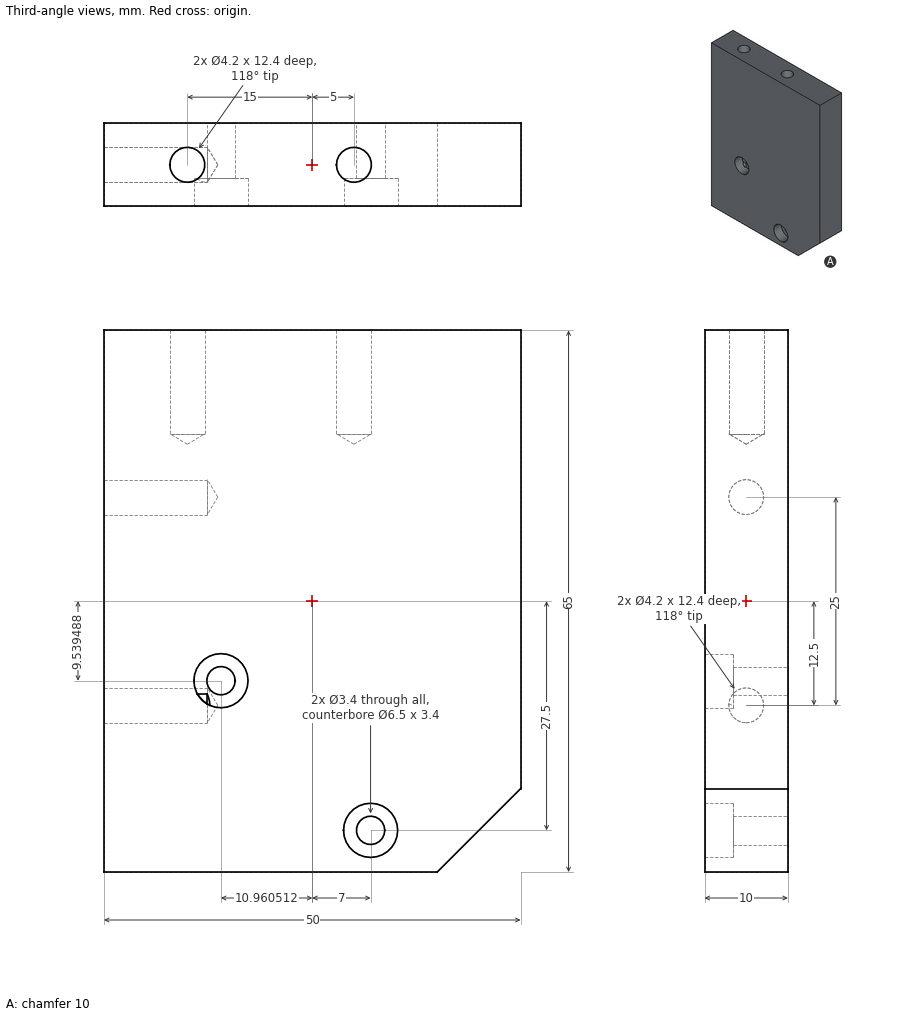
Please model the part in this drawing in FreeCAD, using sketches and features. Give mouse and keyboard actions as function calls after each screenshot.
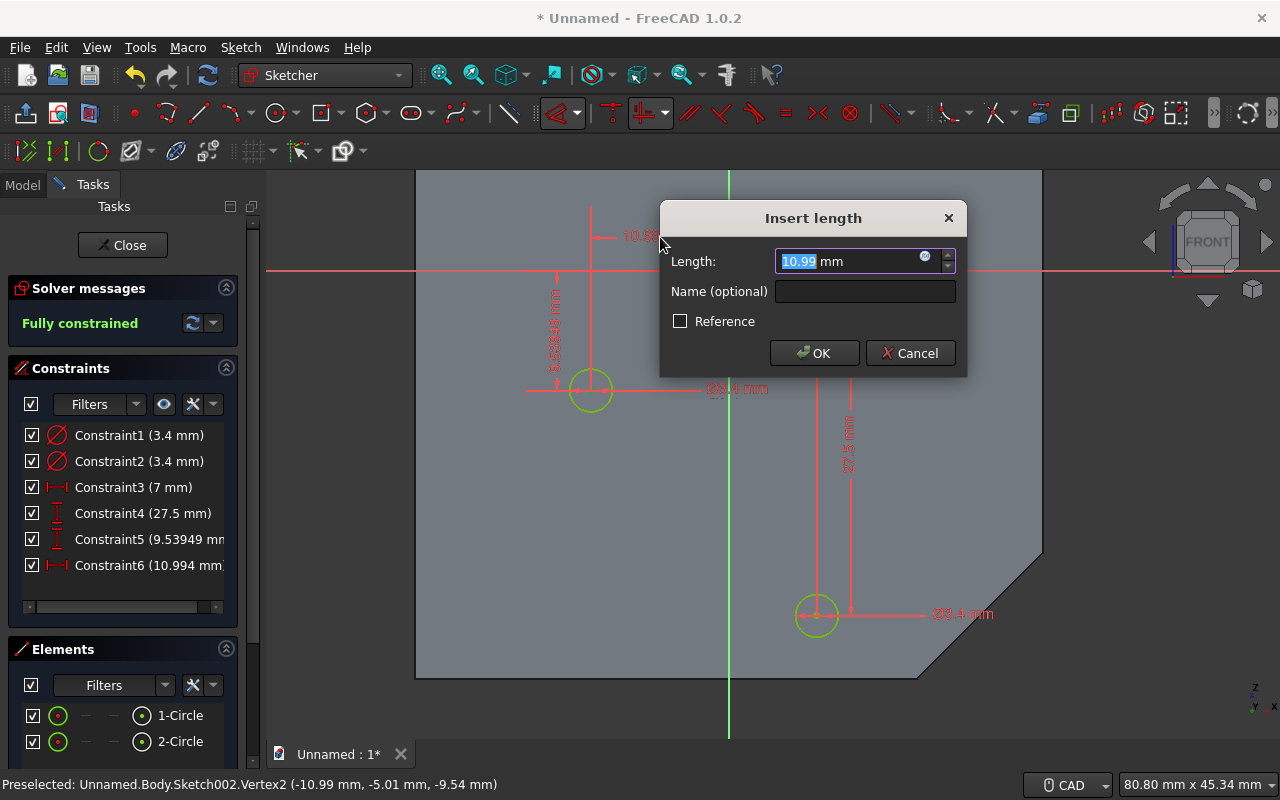
text(10.960512)
key(Return)
key(Escape)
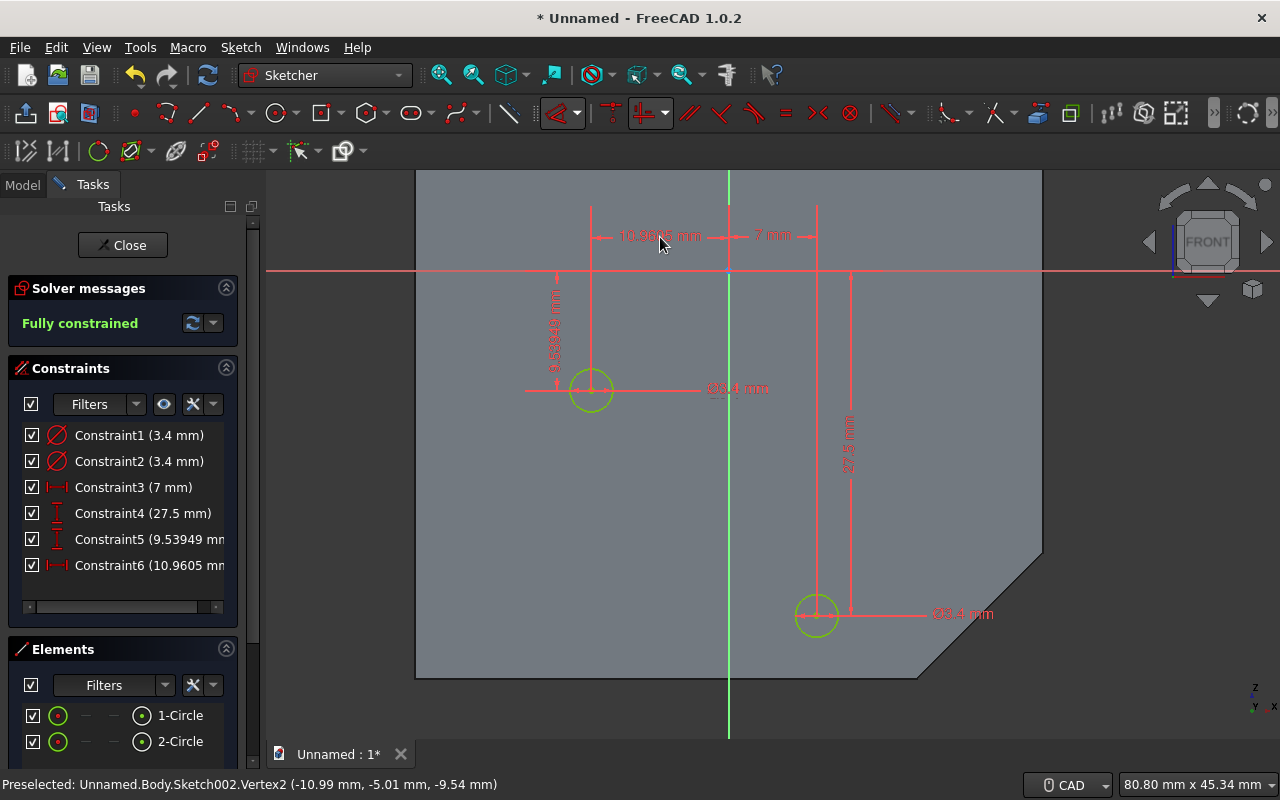
click(123, 245)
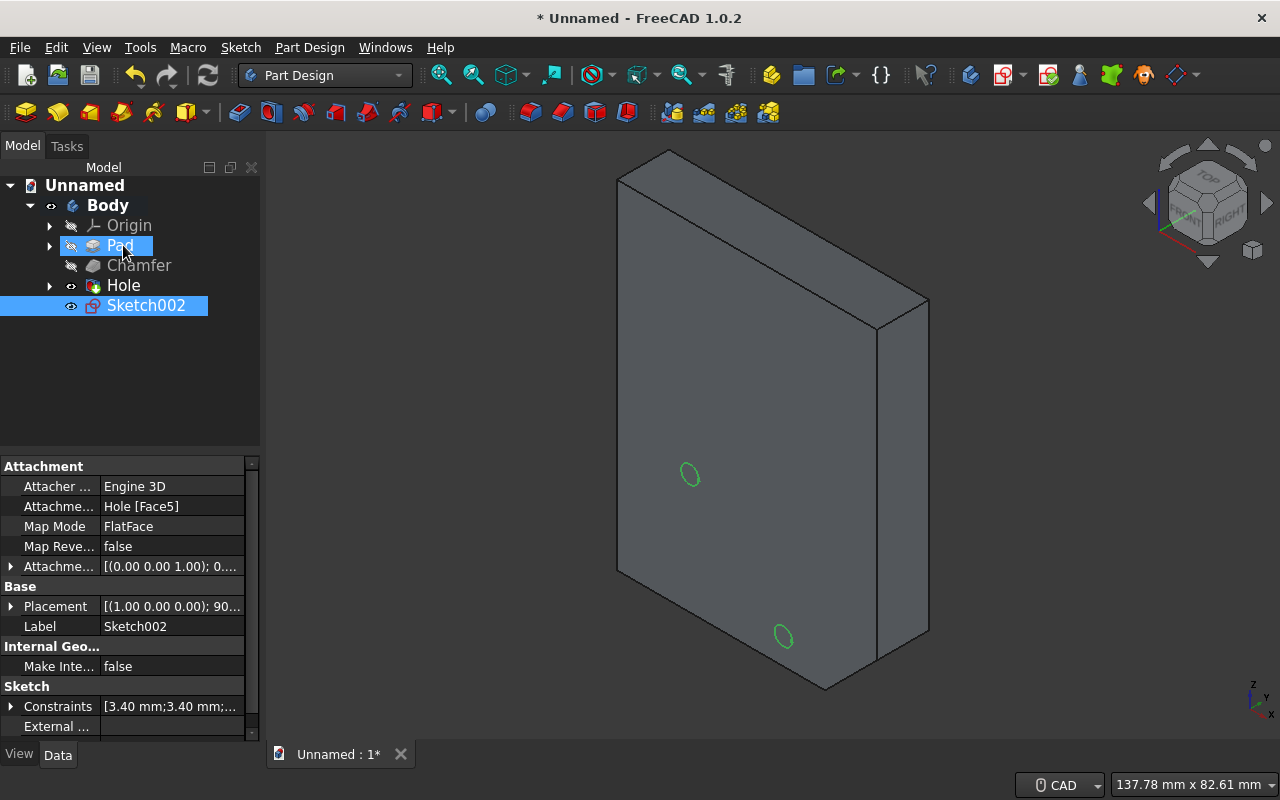
click(272, 112)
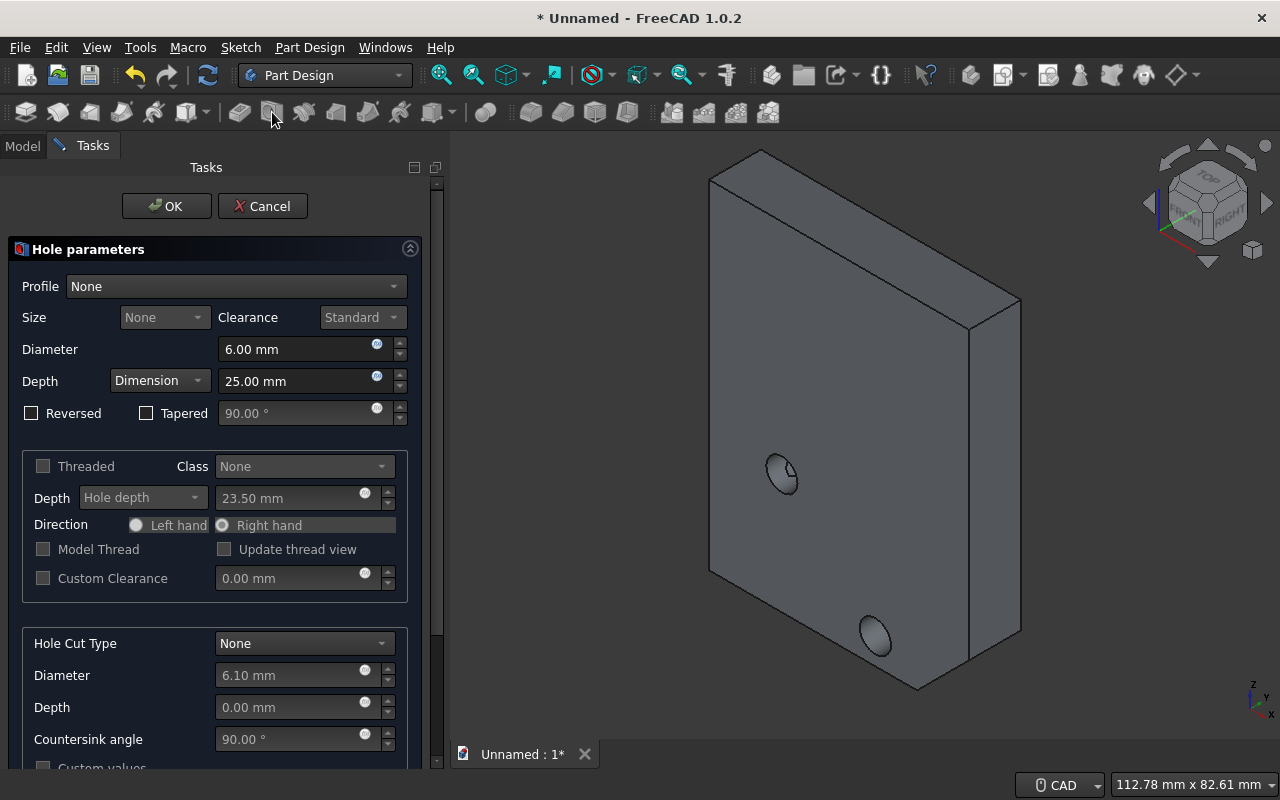
triple_click(305, 349)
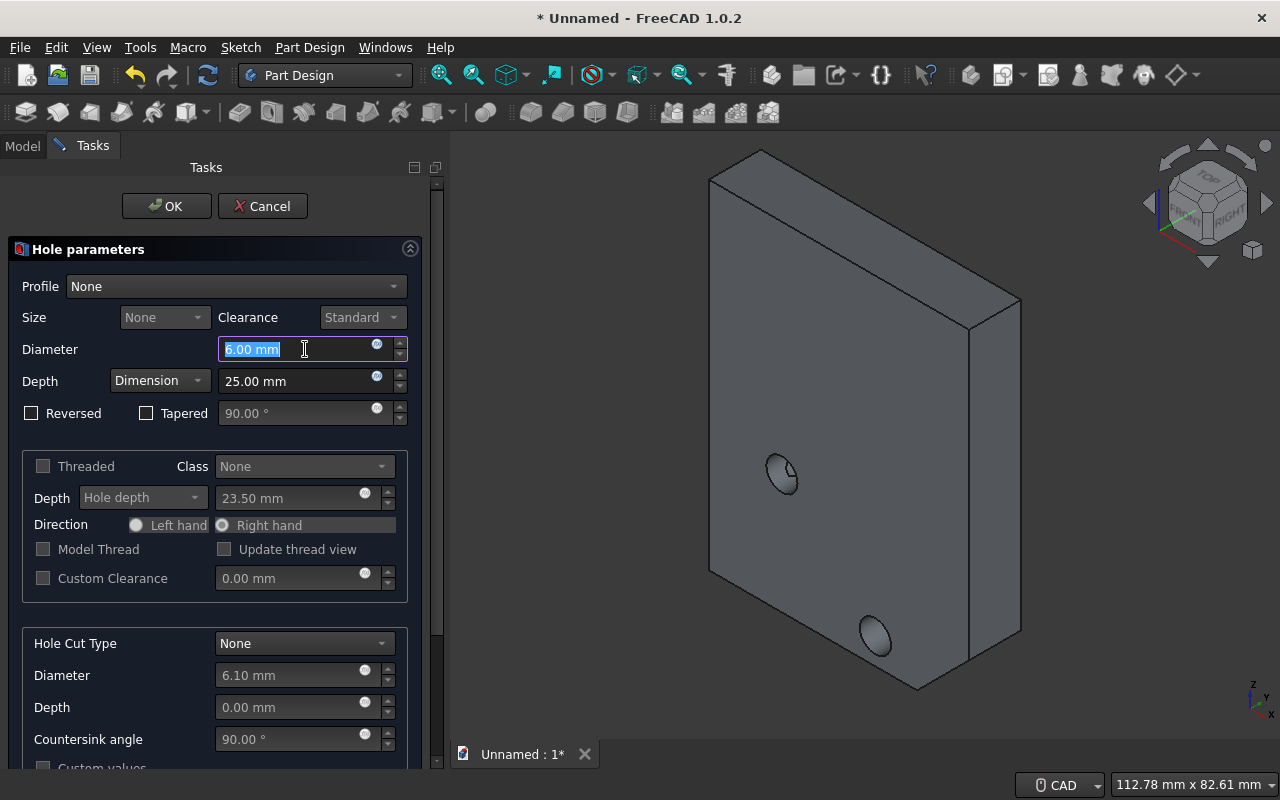
text(3.4)
key(Tab)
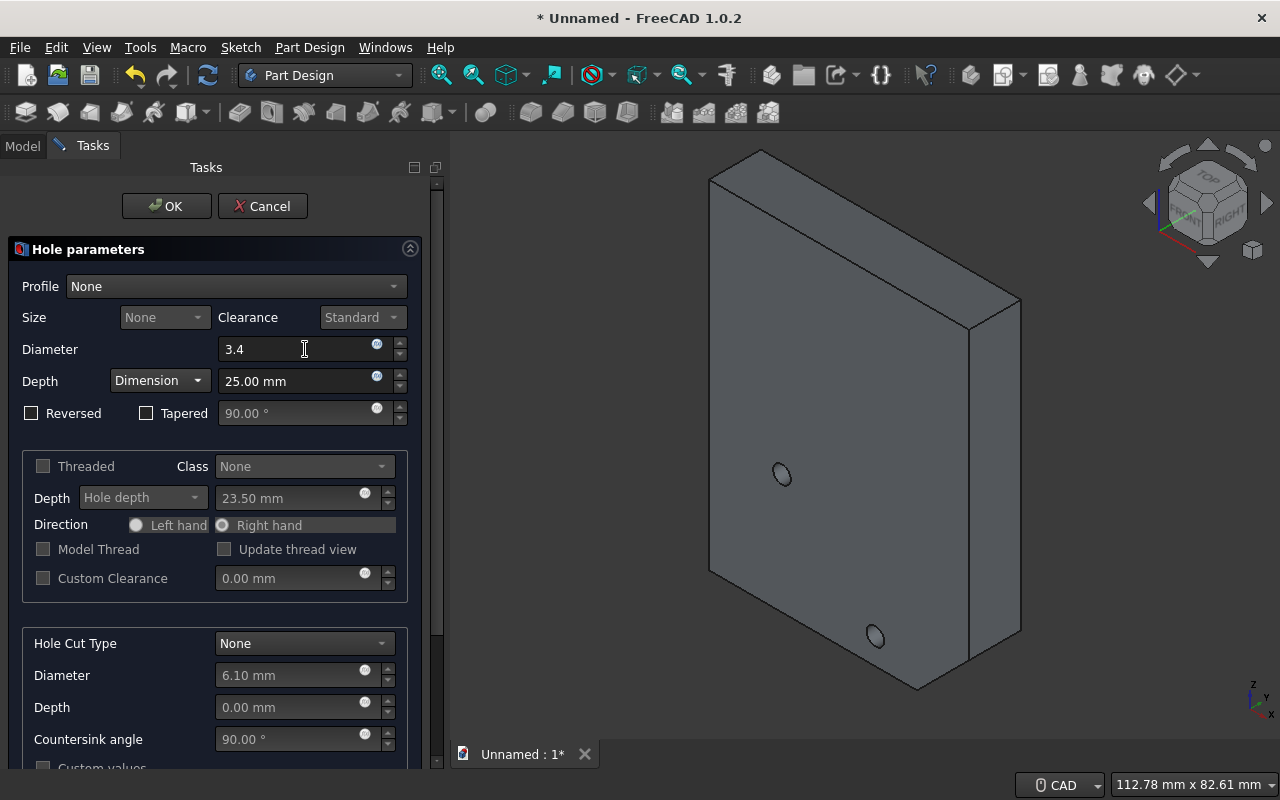
click(161, 380)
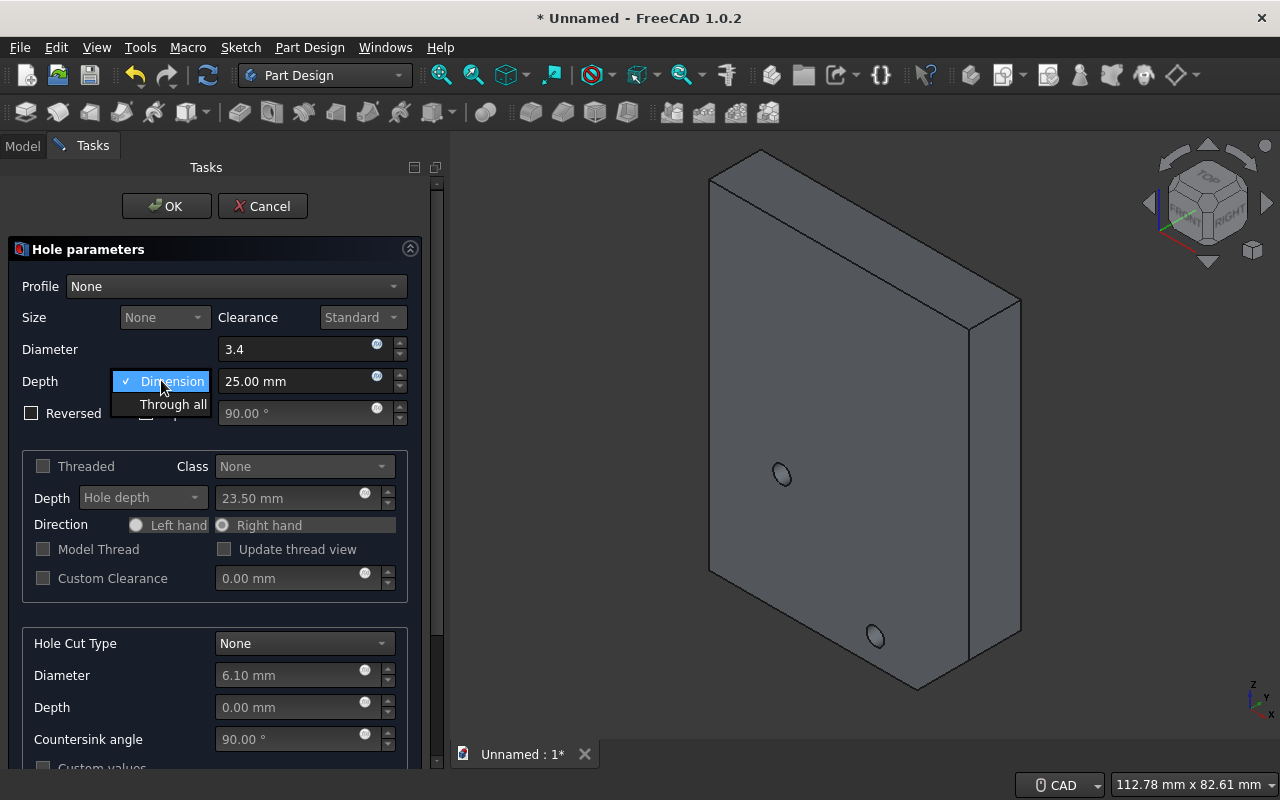
click(160, 404)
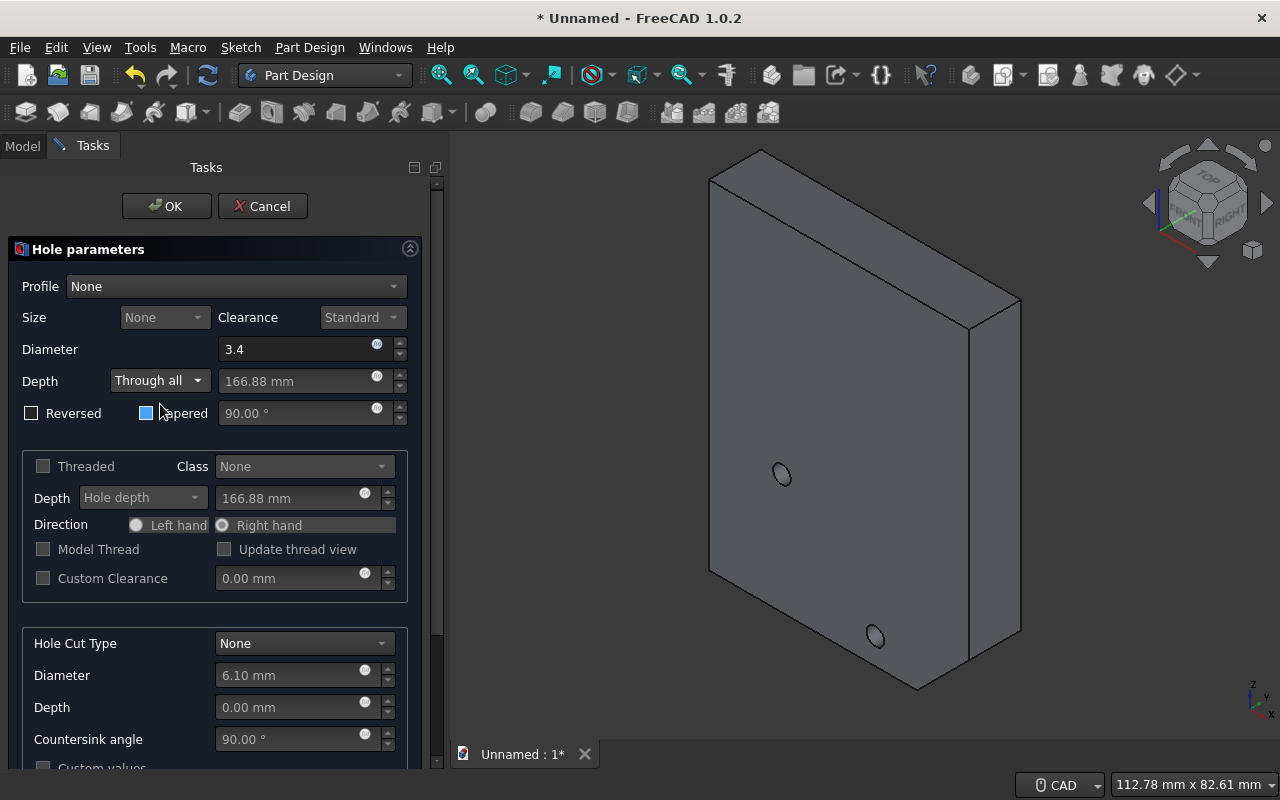
click(306, 644)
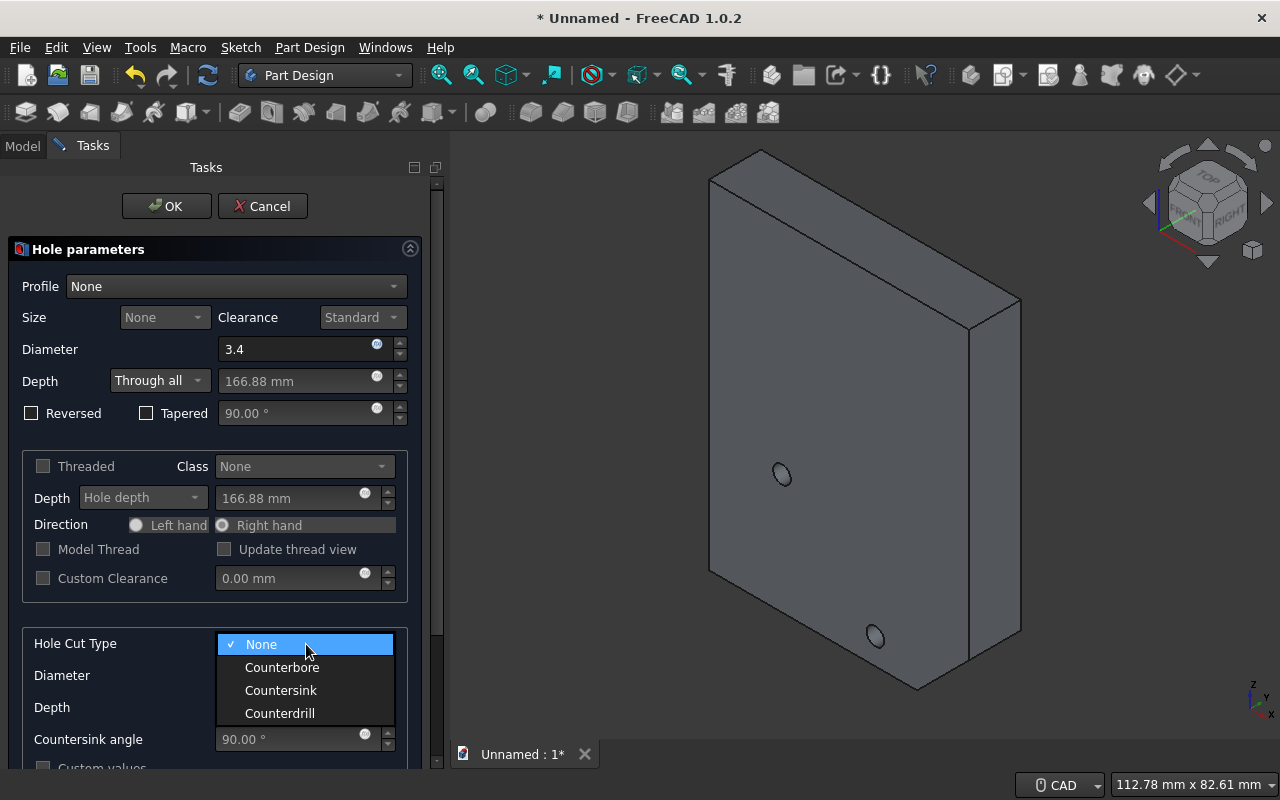
click(304, 668)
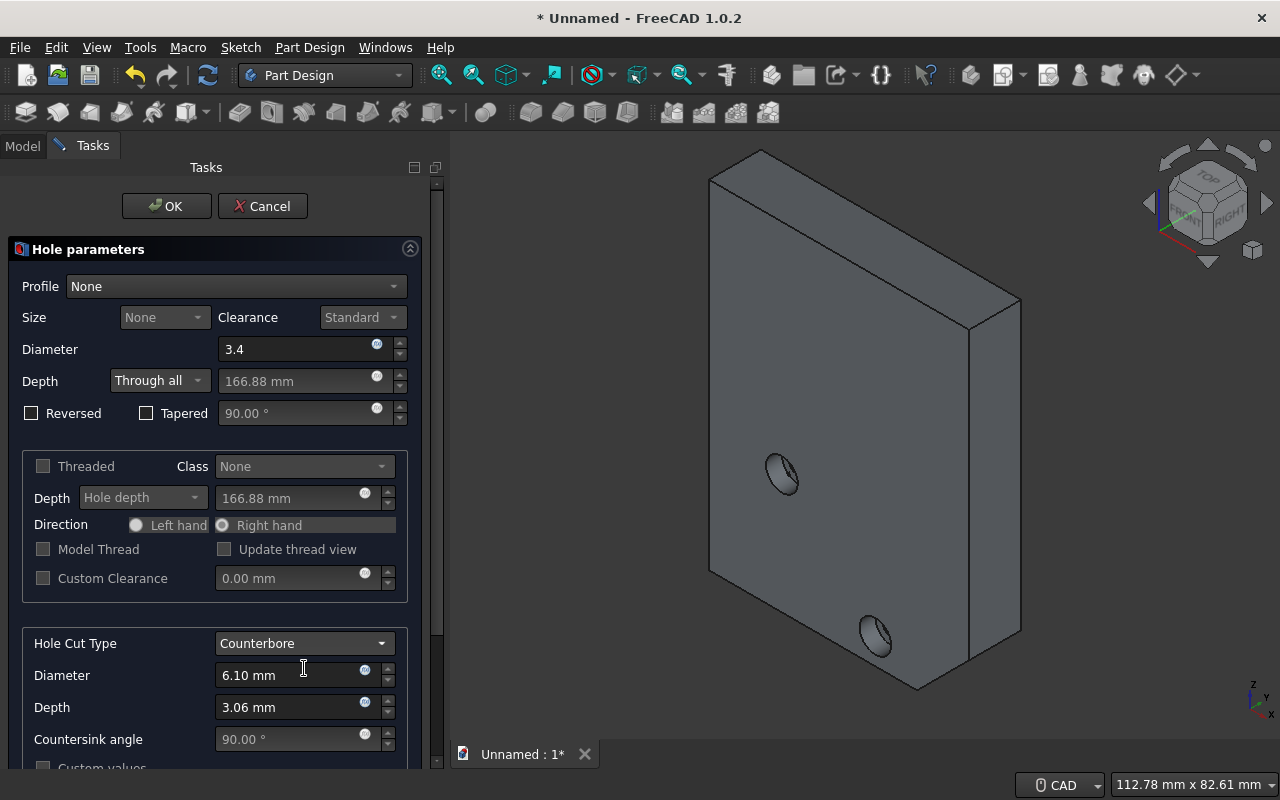
triple_click(298, 675)